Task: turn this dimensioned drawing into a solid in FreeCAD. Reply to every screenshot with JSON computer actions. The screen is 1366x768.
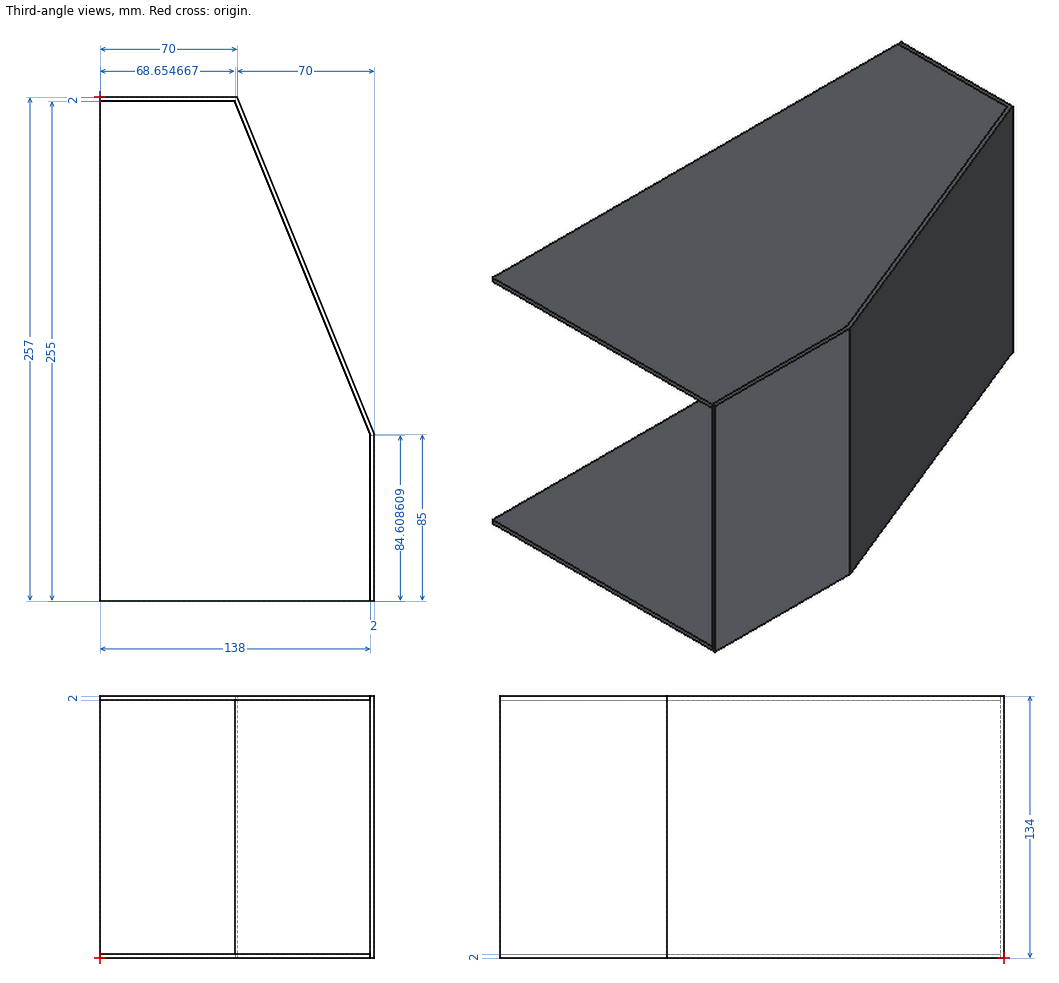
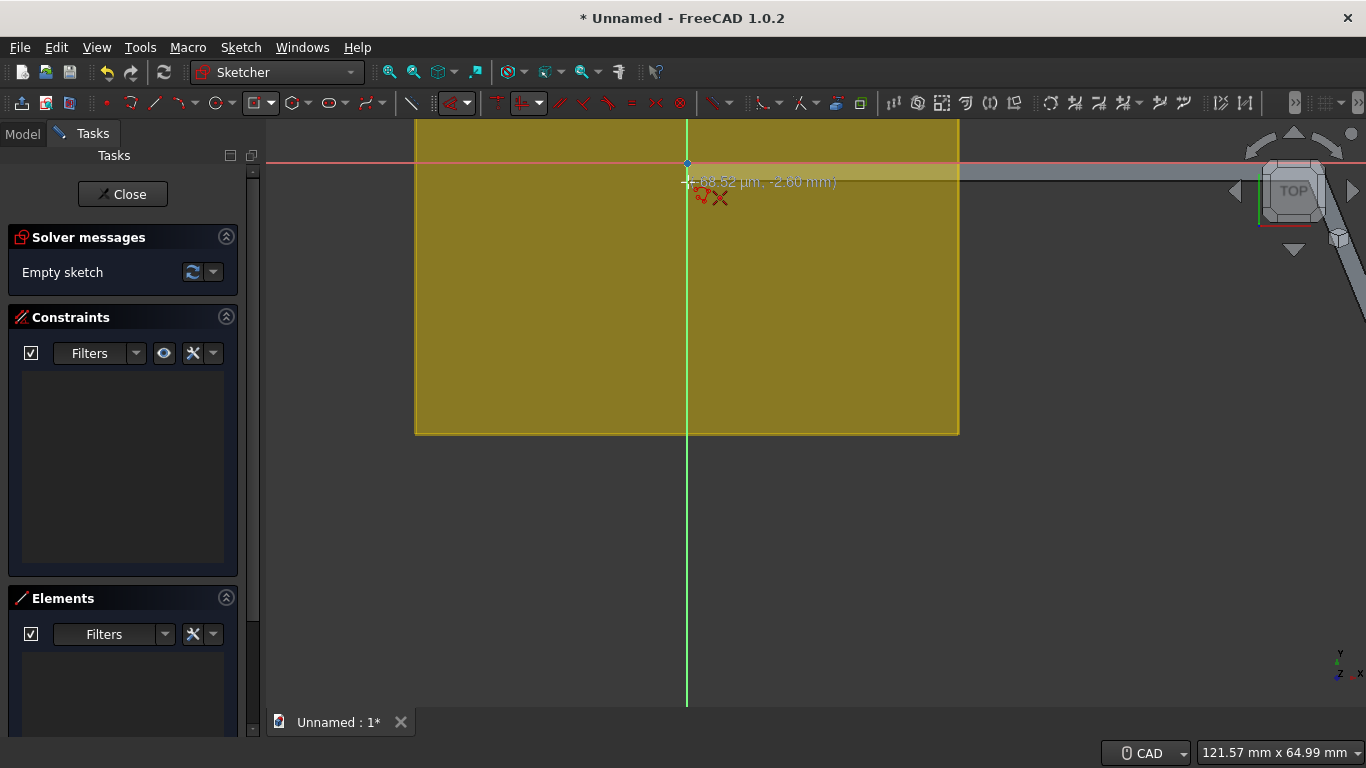
{"action": "left_click", "coordinate": [687, 181]}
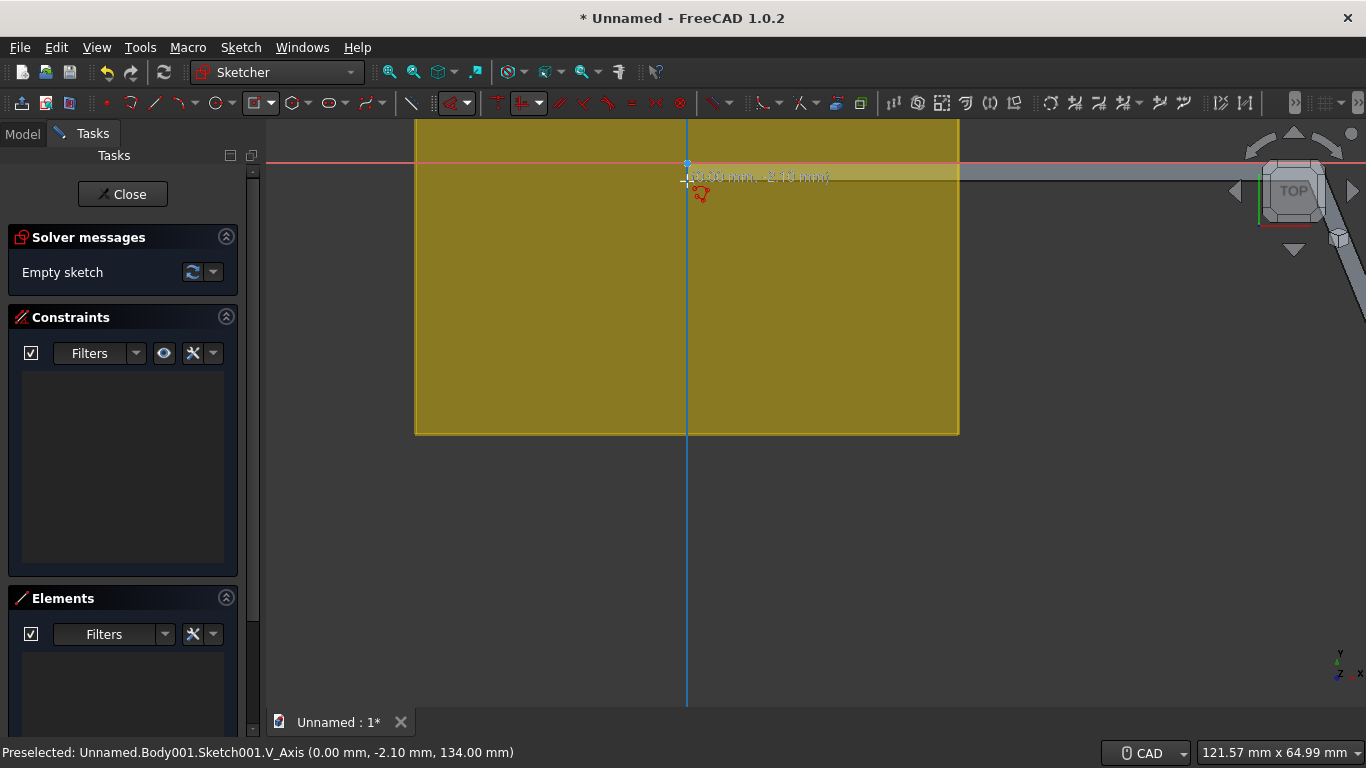
{"action": "scroll", "coordinate": [636, 232], "scroll_direction": "down", "scroll_amount": 9}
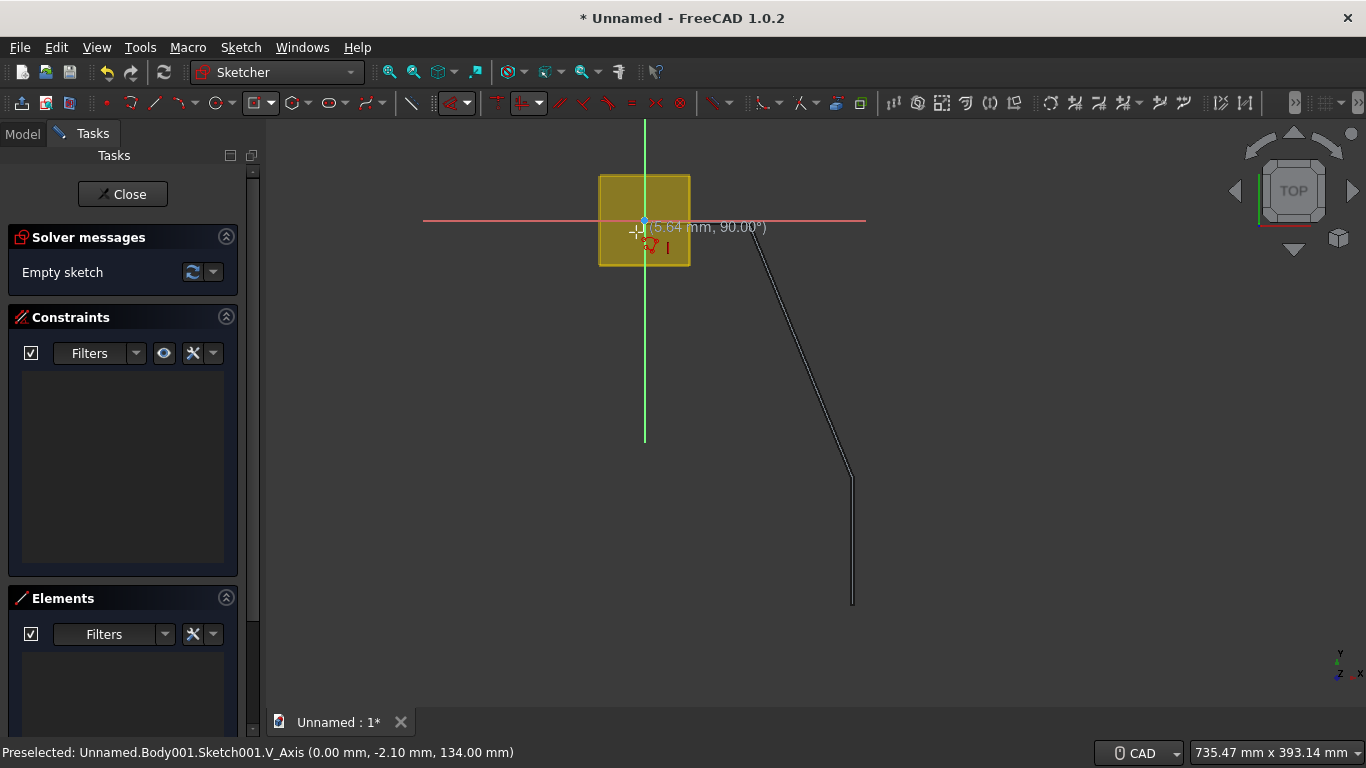
{"action": "left_click", "coordinate": [654, 605]}
{"action": "left_click", "coordinate": [851, 605]}
{"action": "left_click", "coordinate": [851, 479]}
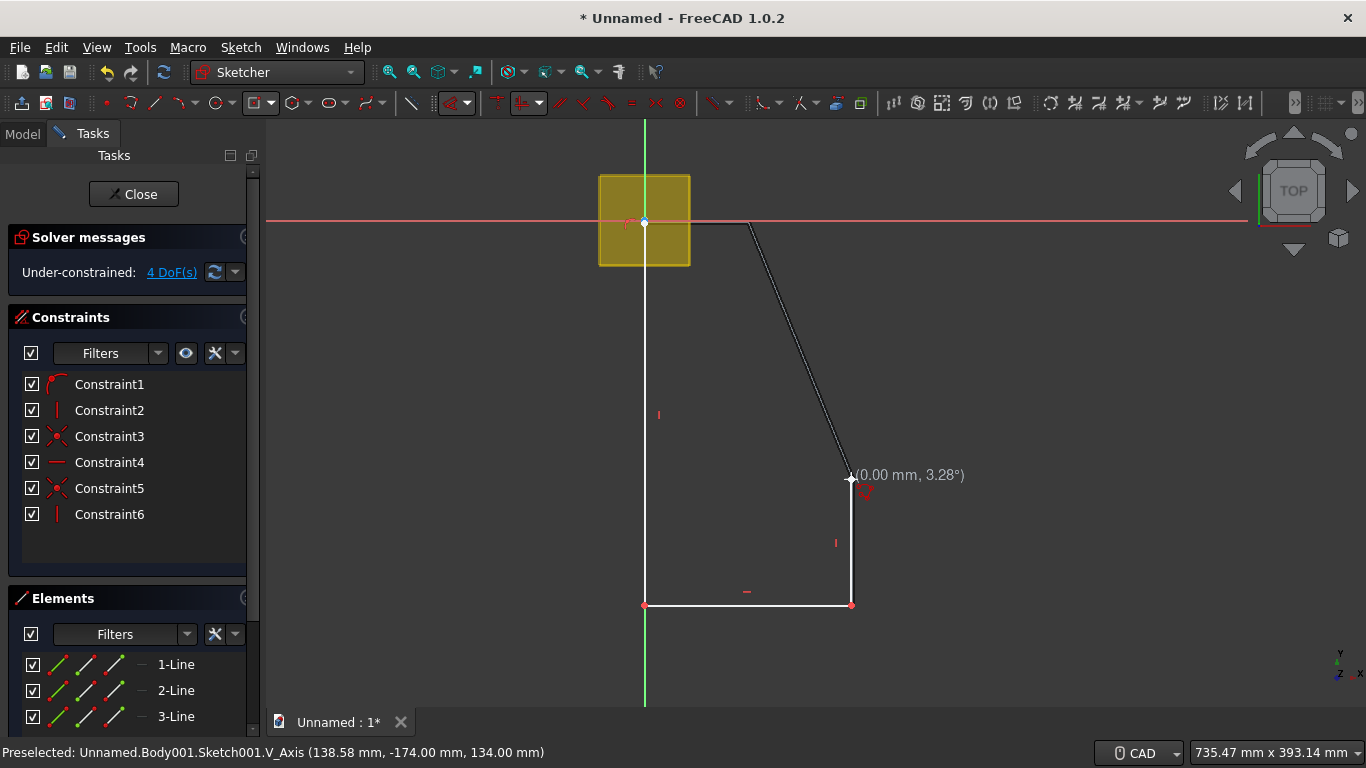
{"action": "scroll", "coordinate": [747, 224], "scroll_direction": "up", "scroll_amount": 9}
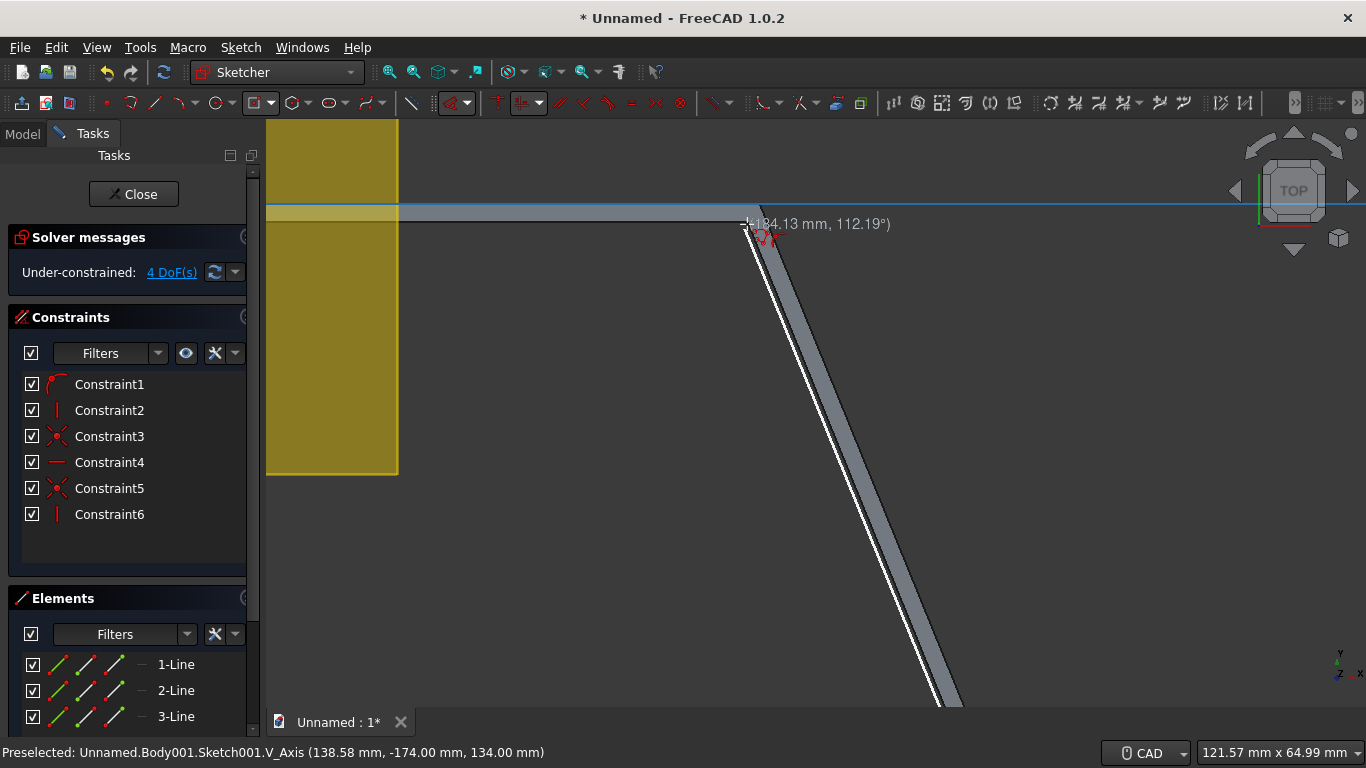
{"action": "left_click", "coordinate": [747, 222]}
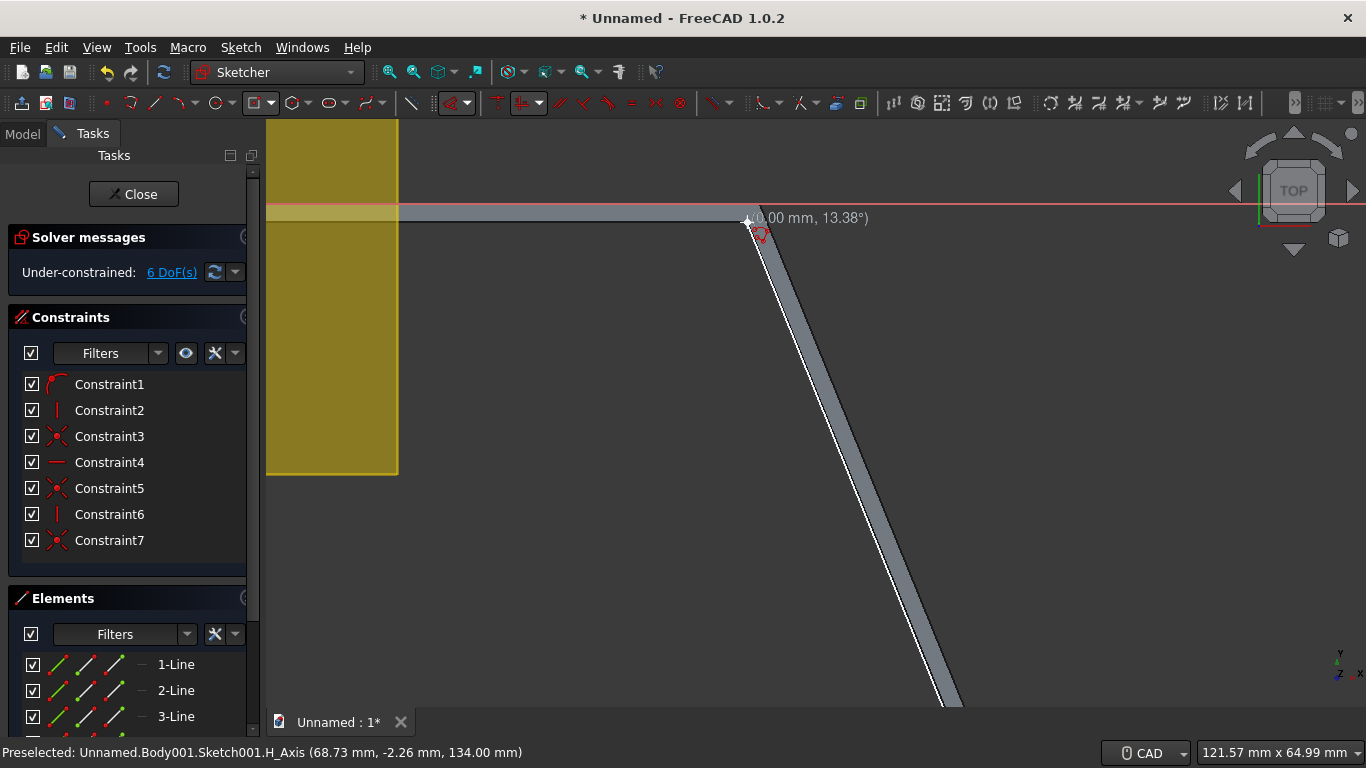
{"action": "scroll", "coordinate": [747, 224], "scroll_direction": "down", "scroll_amount": 9}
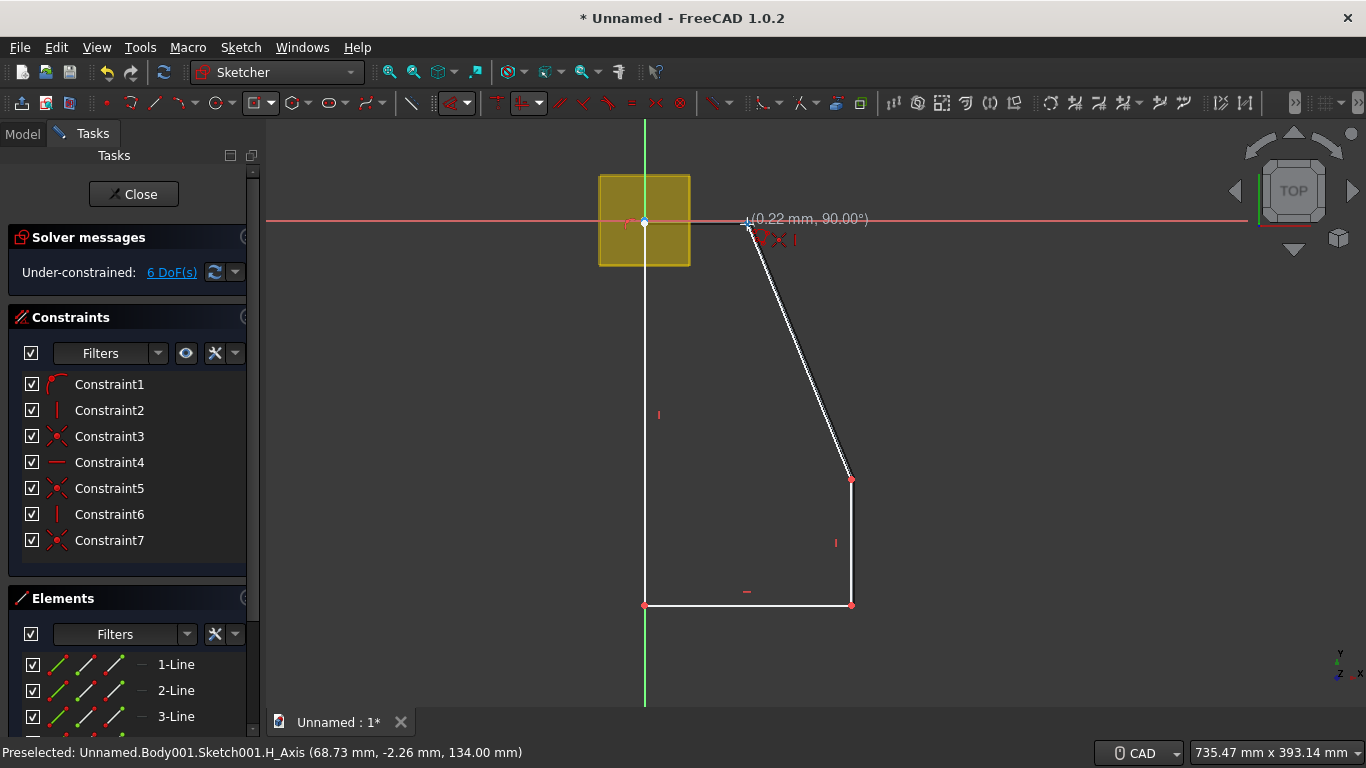
{"action": "scroll", "coordinate": [645, 224], "scroll_direction": "up", "scroll_amount": 9}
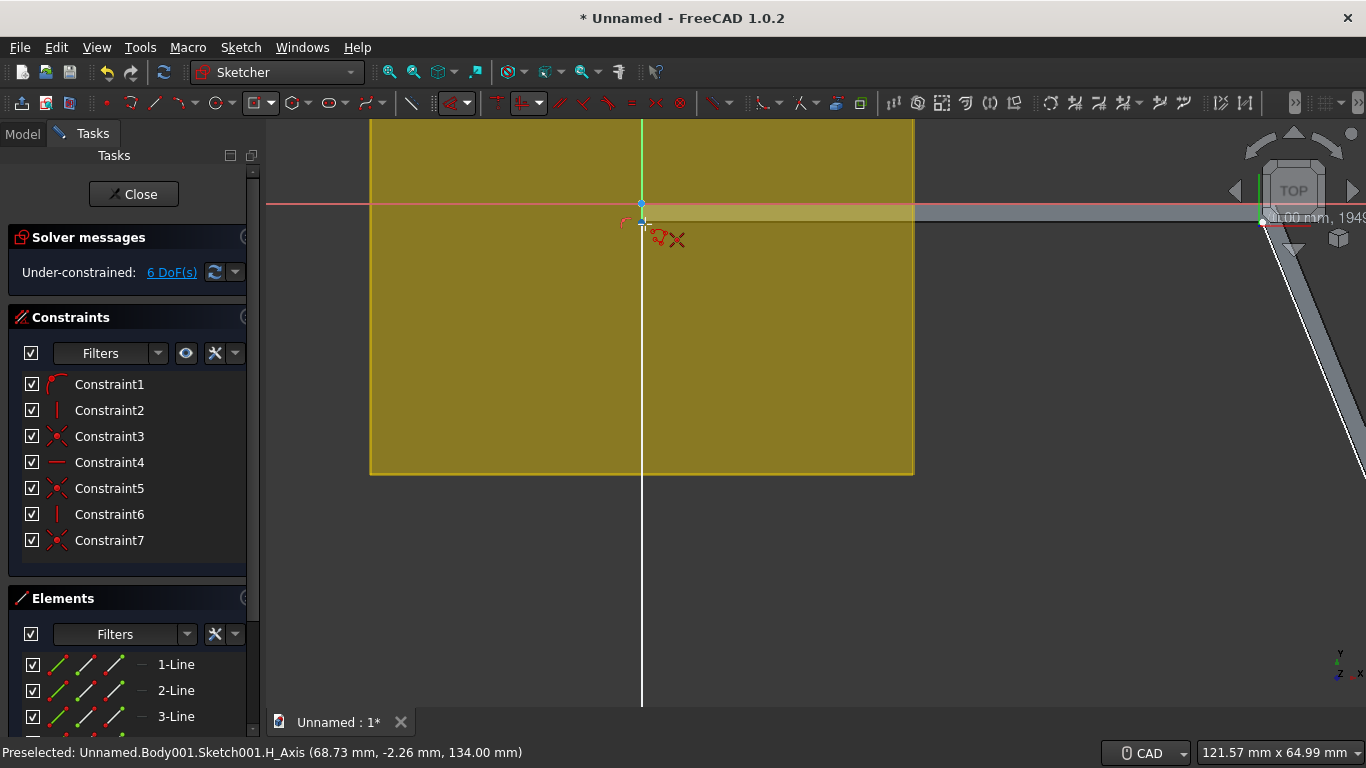
{"action": "left_click", "coordinate": [642, 222]}
{"action": "key", "text": "Escape"}
{"action": "key", "text": "Escape"}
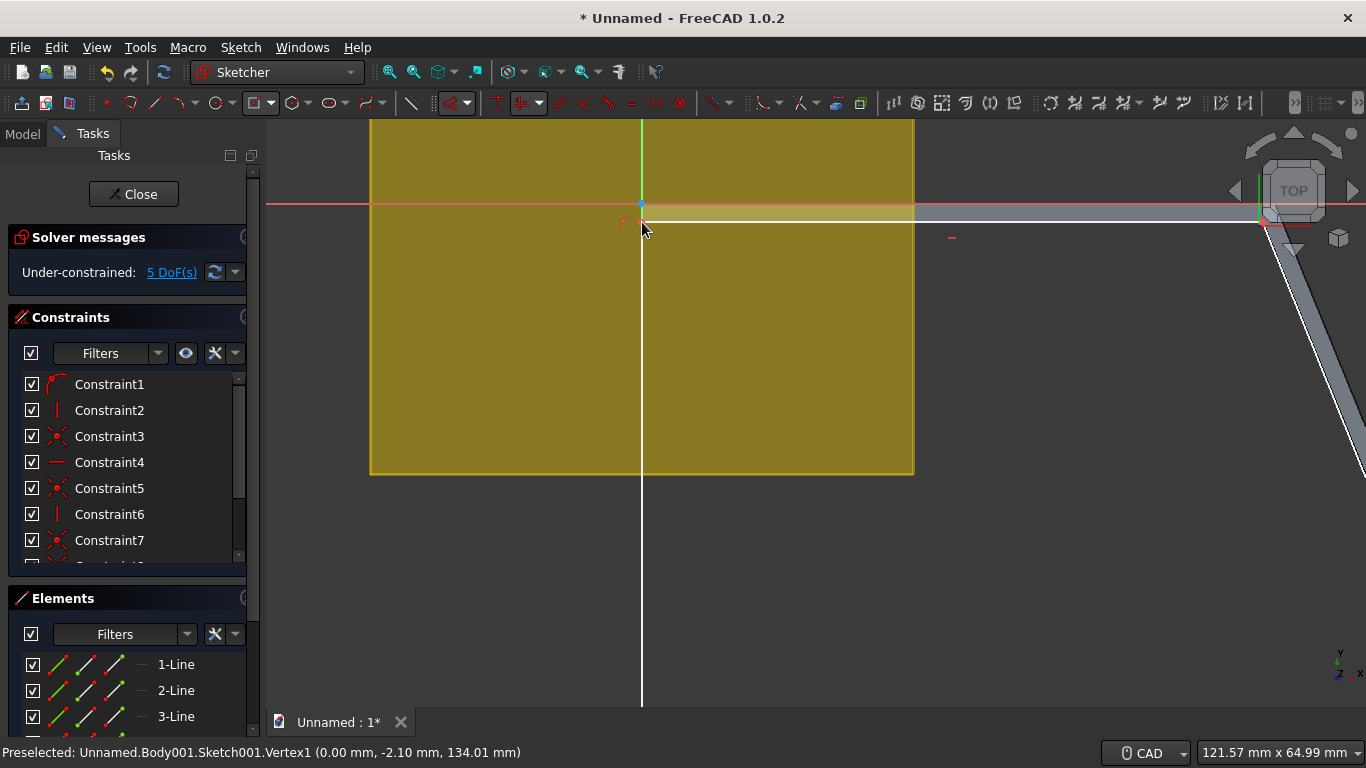
{"action": "key", "text": "d"}